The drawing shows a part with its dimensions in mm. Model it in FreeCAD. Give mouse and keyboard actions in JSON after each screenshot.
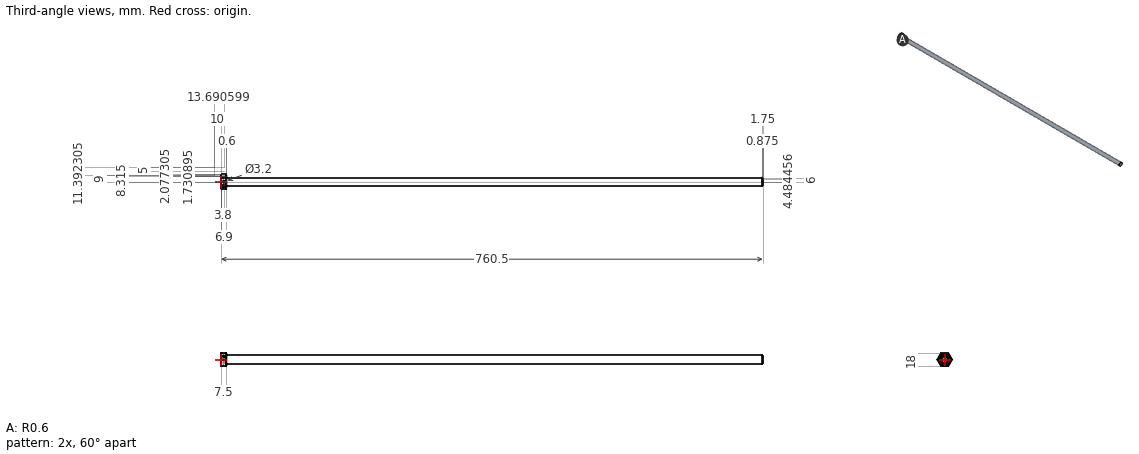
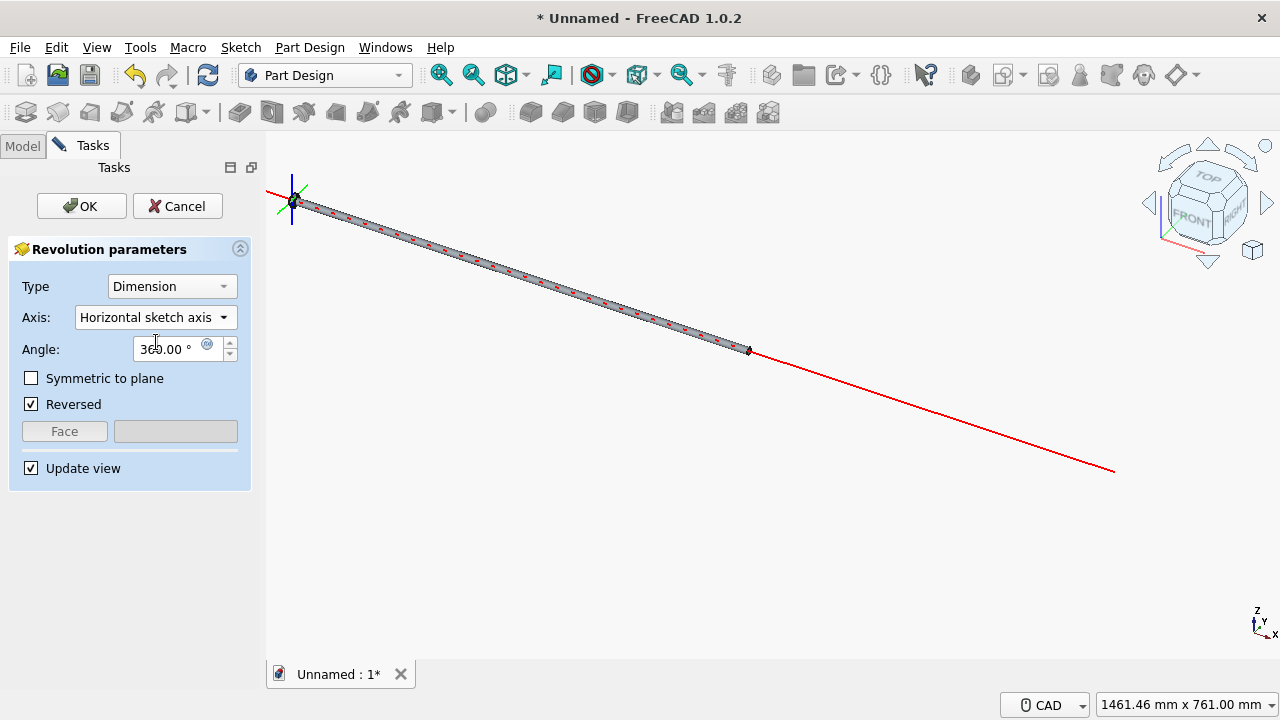
{"action": "left_click", "coordinate": [82, 206]}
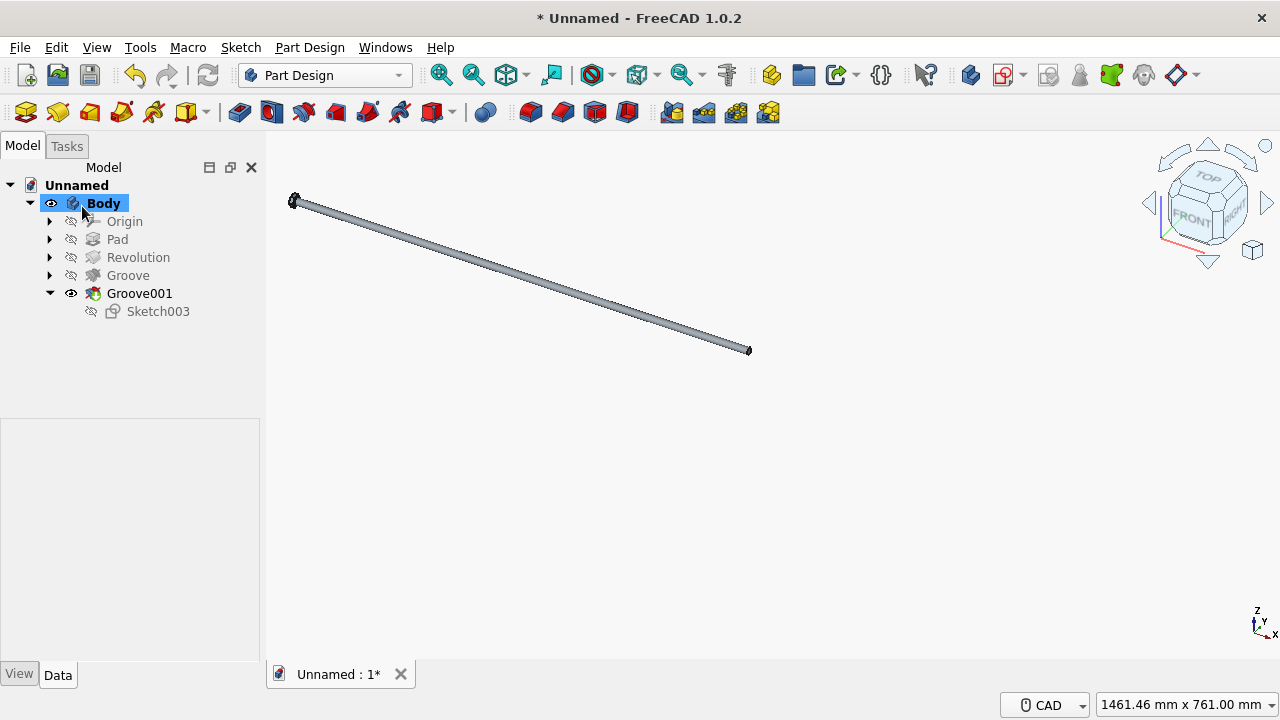
{"action": "key", "text": "0"}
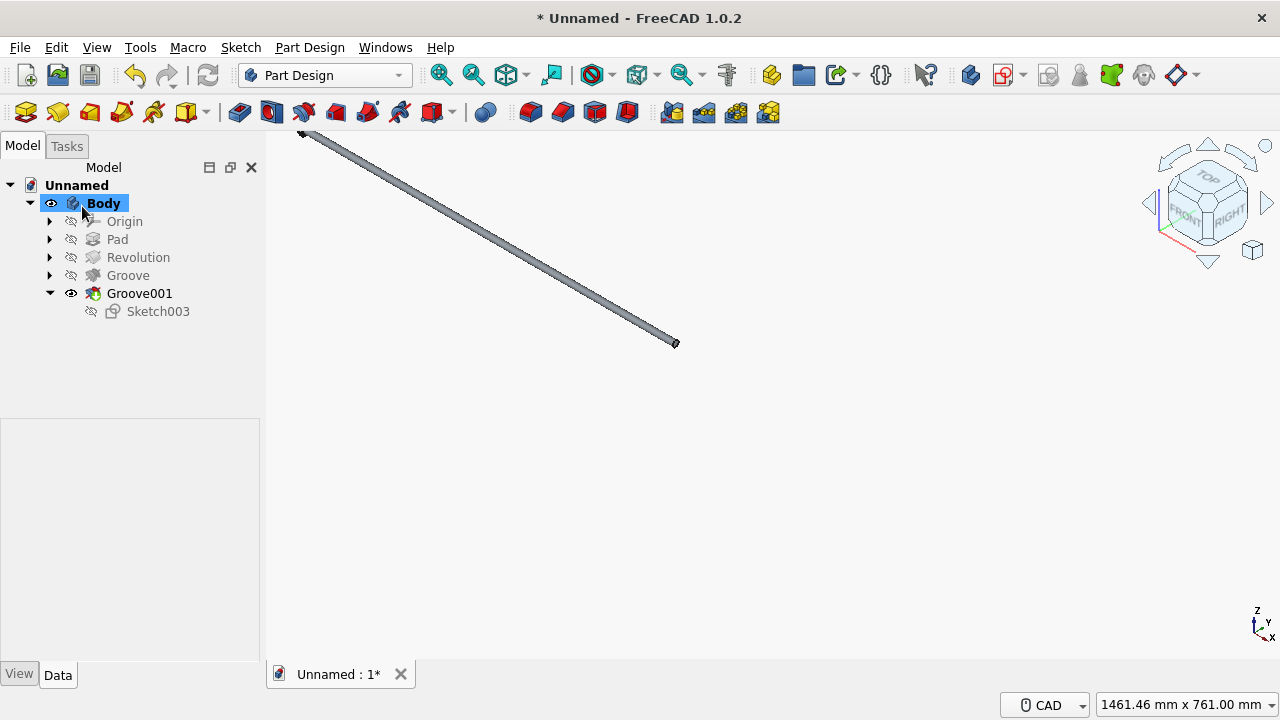
{"action": "key", "text": "v f"}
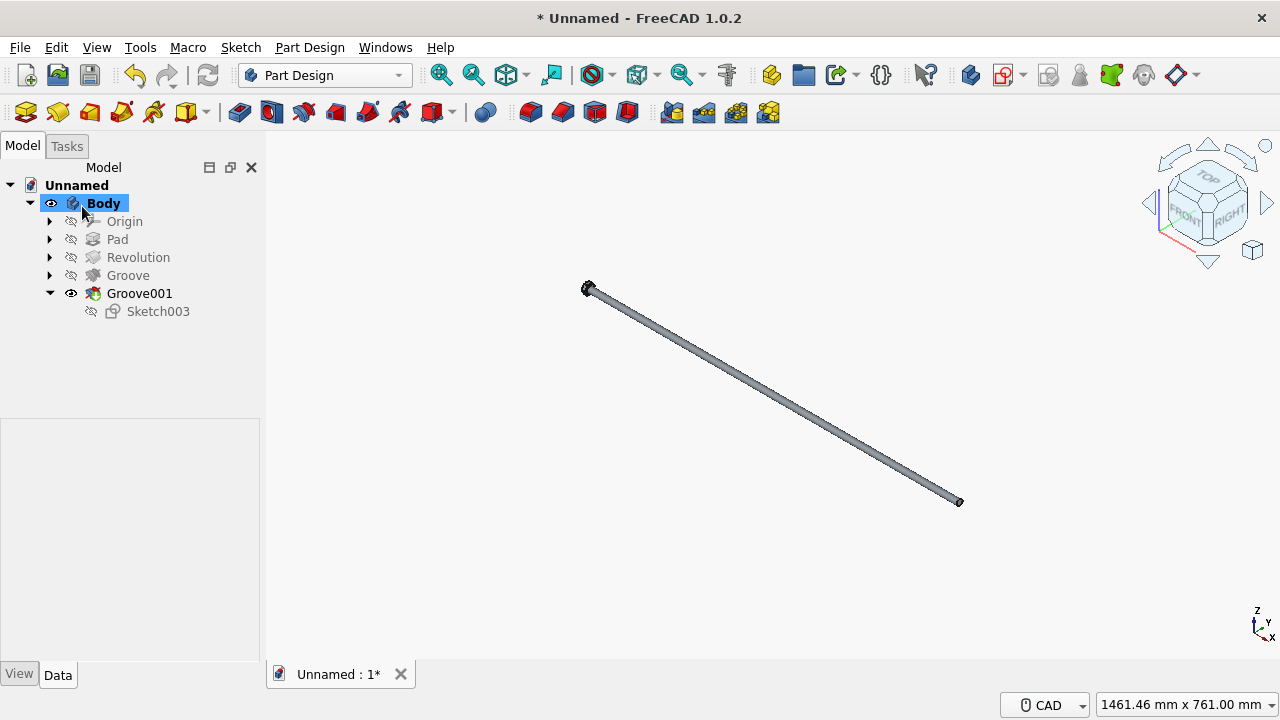
{"action": "key", "text": "2"}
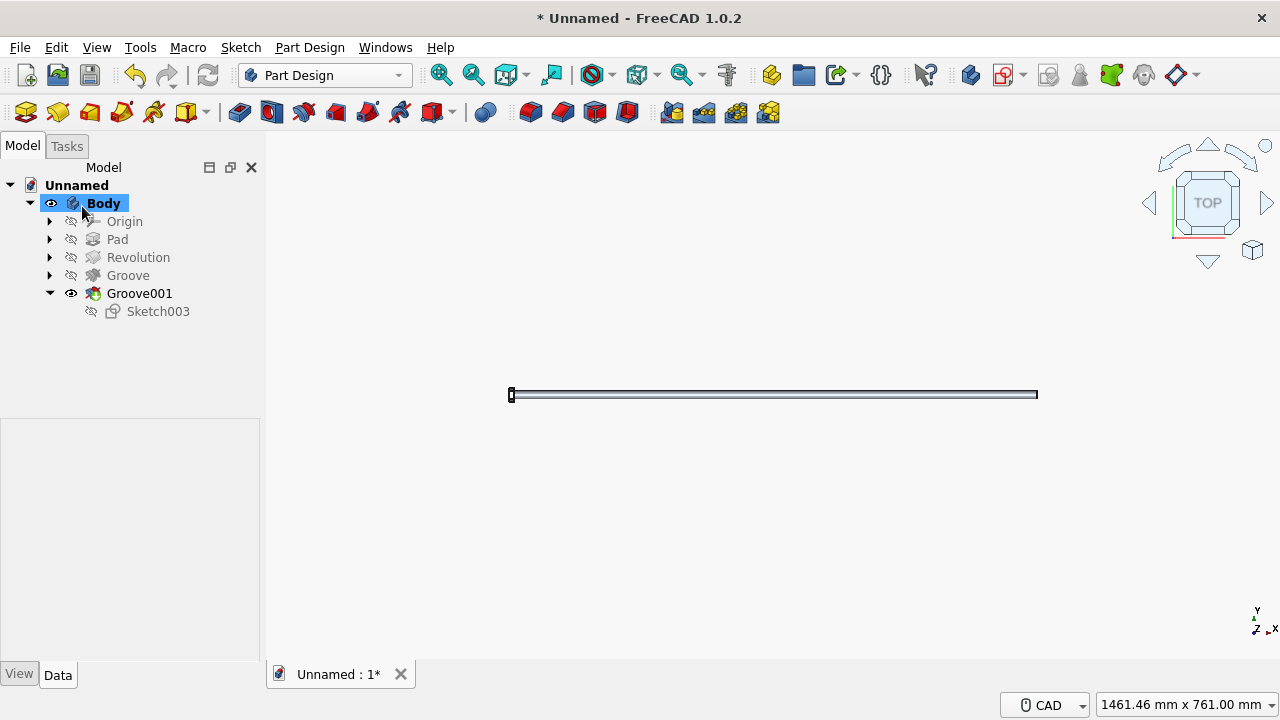
{"action": "key", "text": "1"}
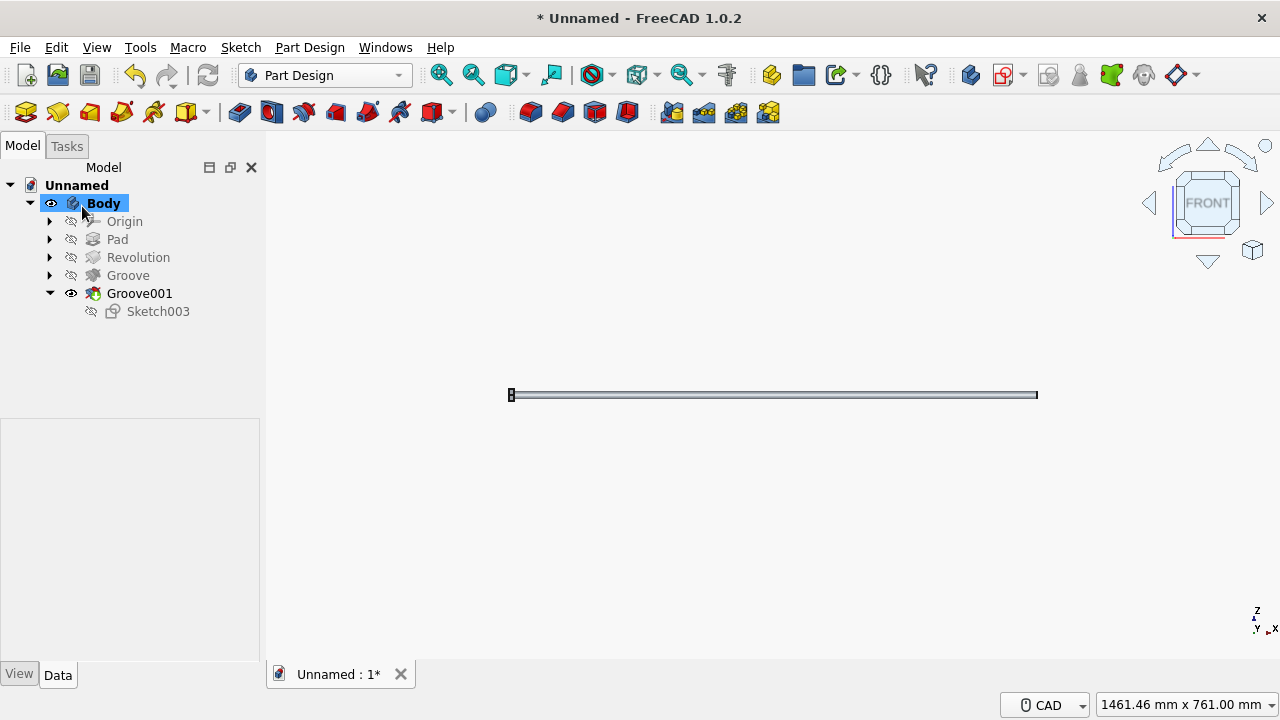
{"action": "key", "text": "3"}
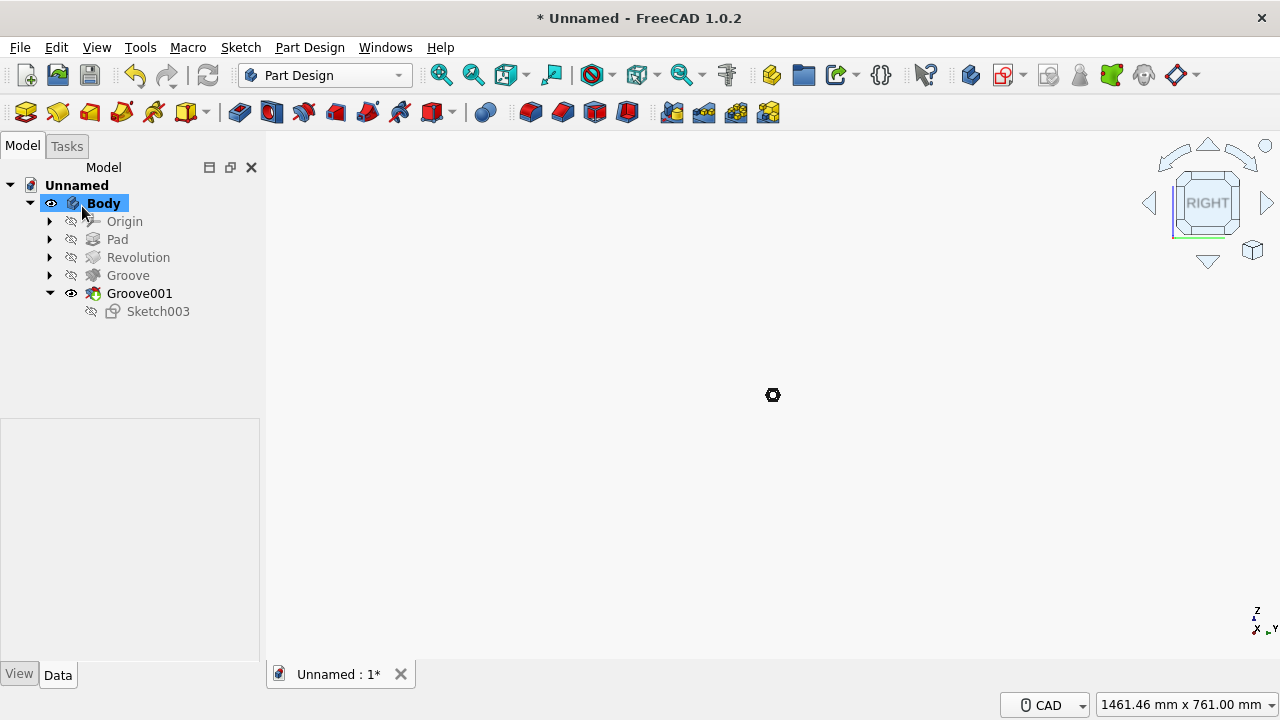
{"action": "left_click", "coordinate": [442, 76]}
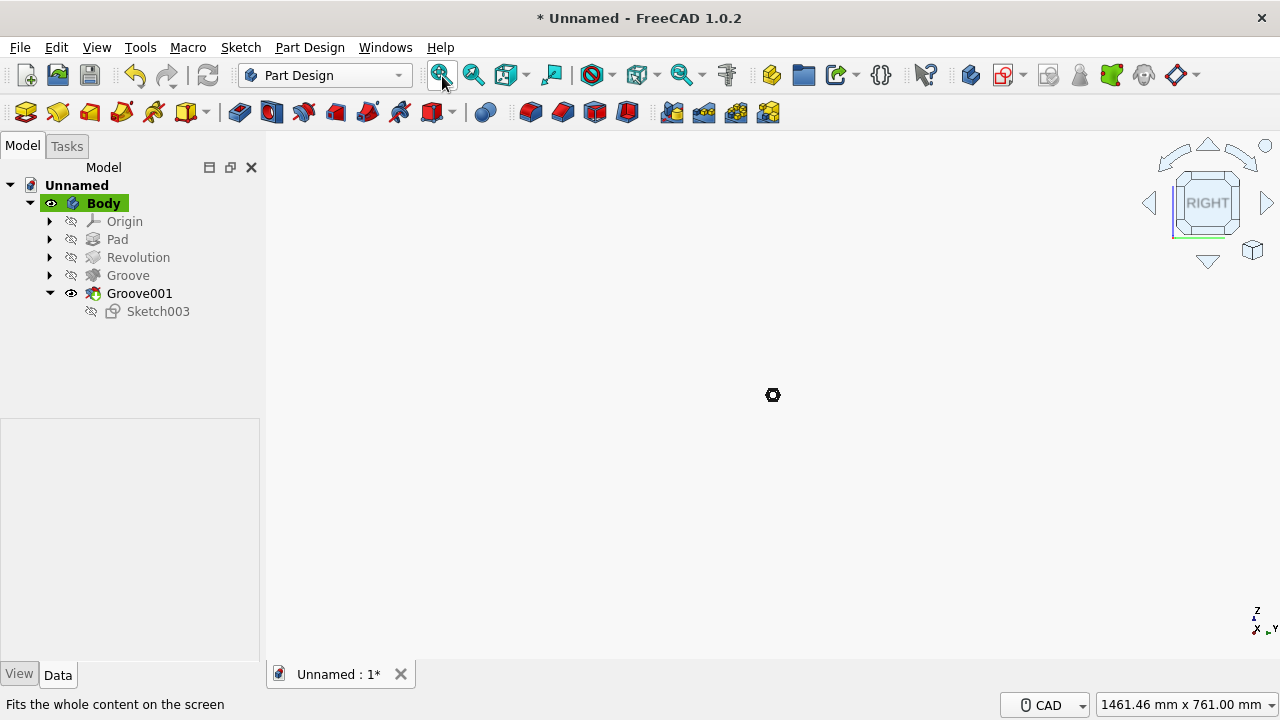
{"action": "key", "text": "5"}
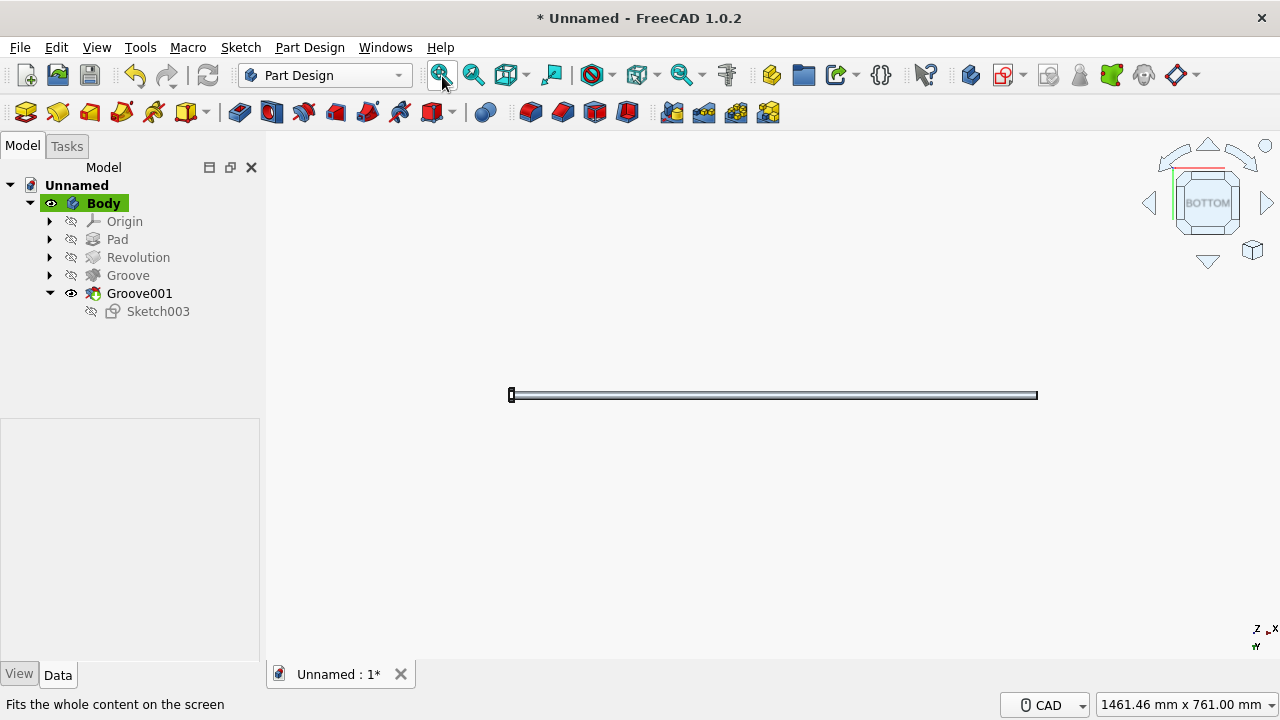
{"action": "key", "text": "4"}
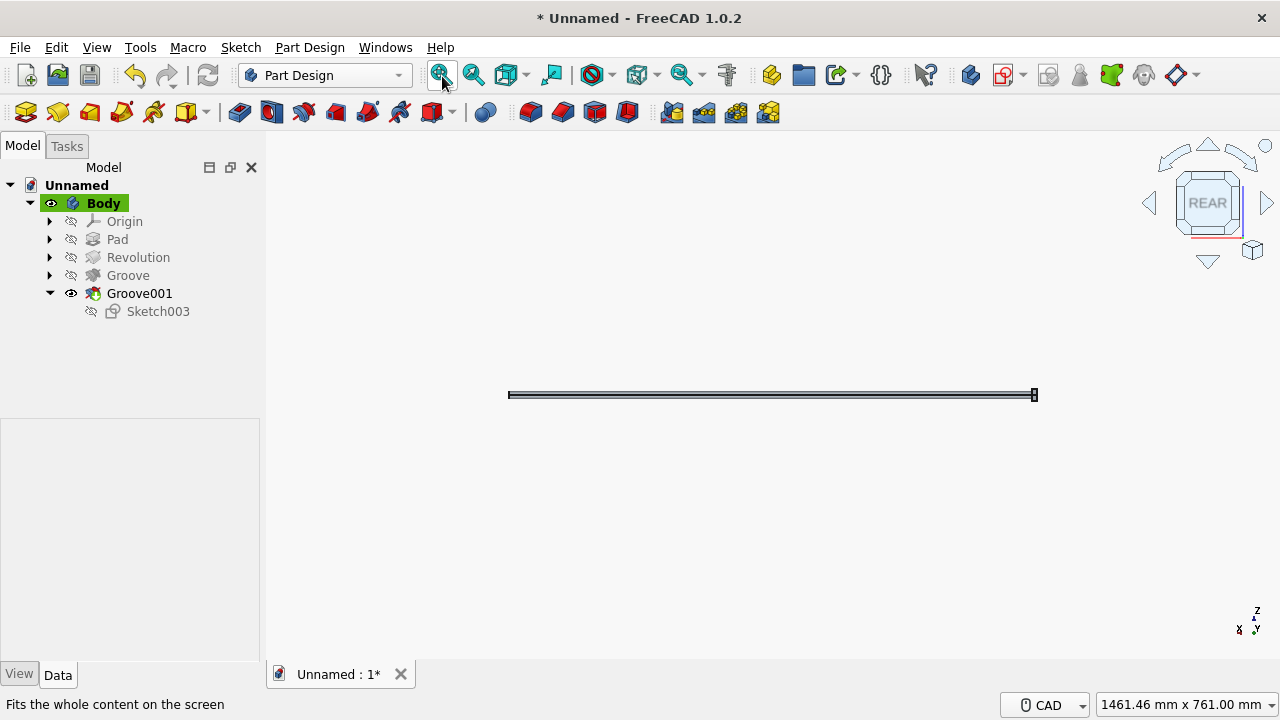
{"action": "key", "text": "6"}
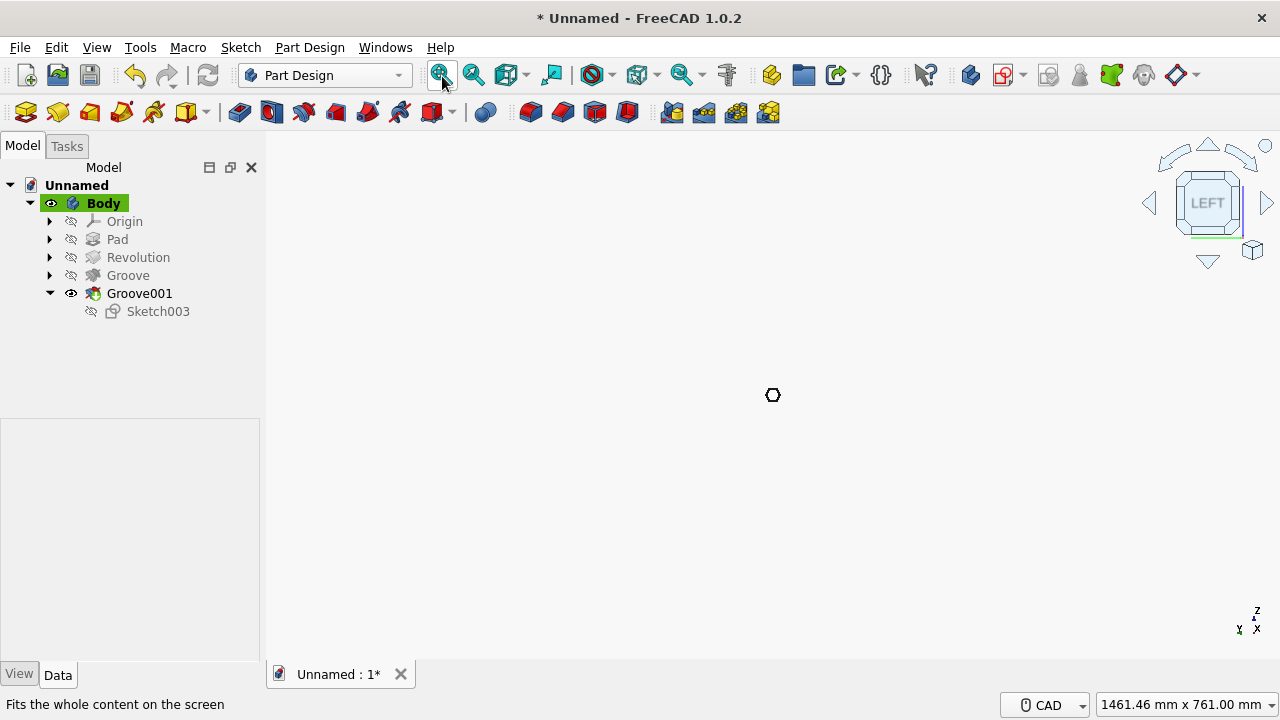
{"action": "left_click", "coordinate": [442, 76]}